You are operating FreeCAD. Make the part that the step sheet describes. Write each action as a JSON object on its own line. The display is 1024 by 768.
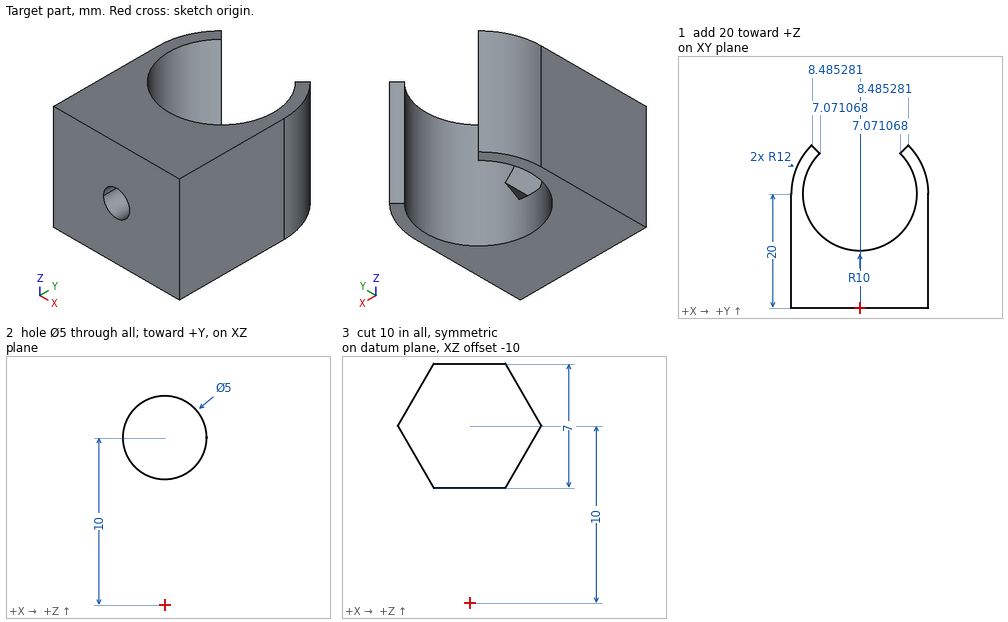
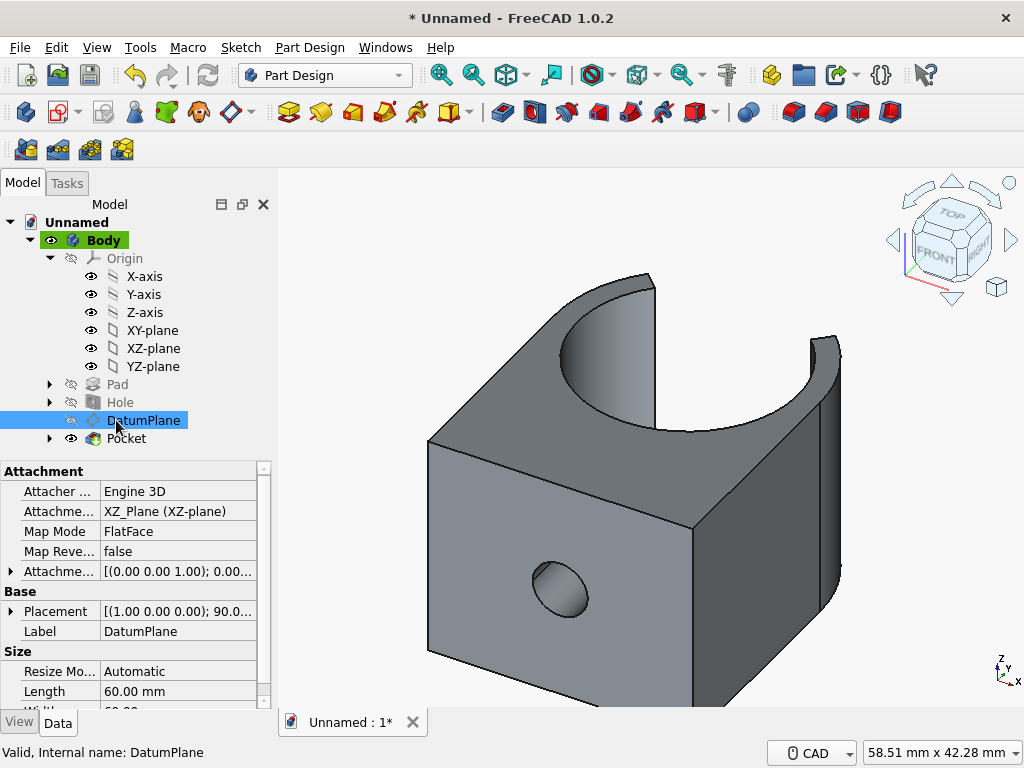
{"action": "key", "text": "0"}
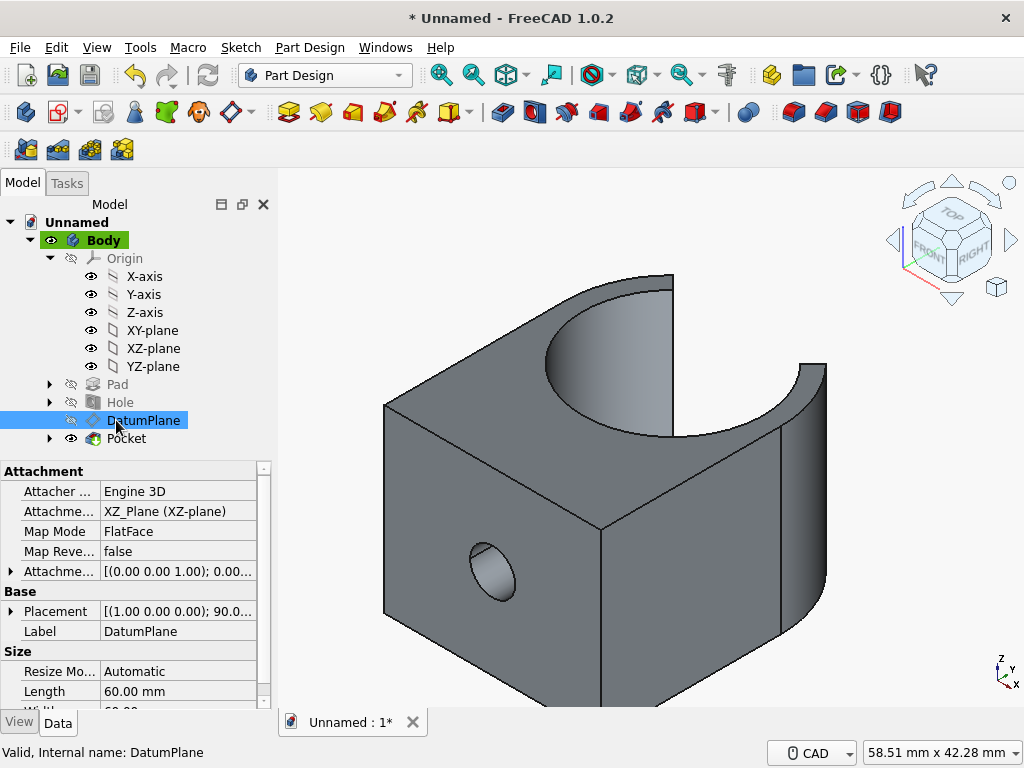
{"action": "left_click", "coordinate": [442, 76]}